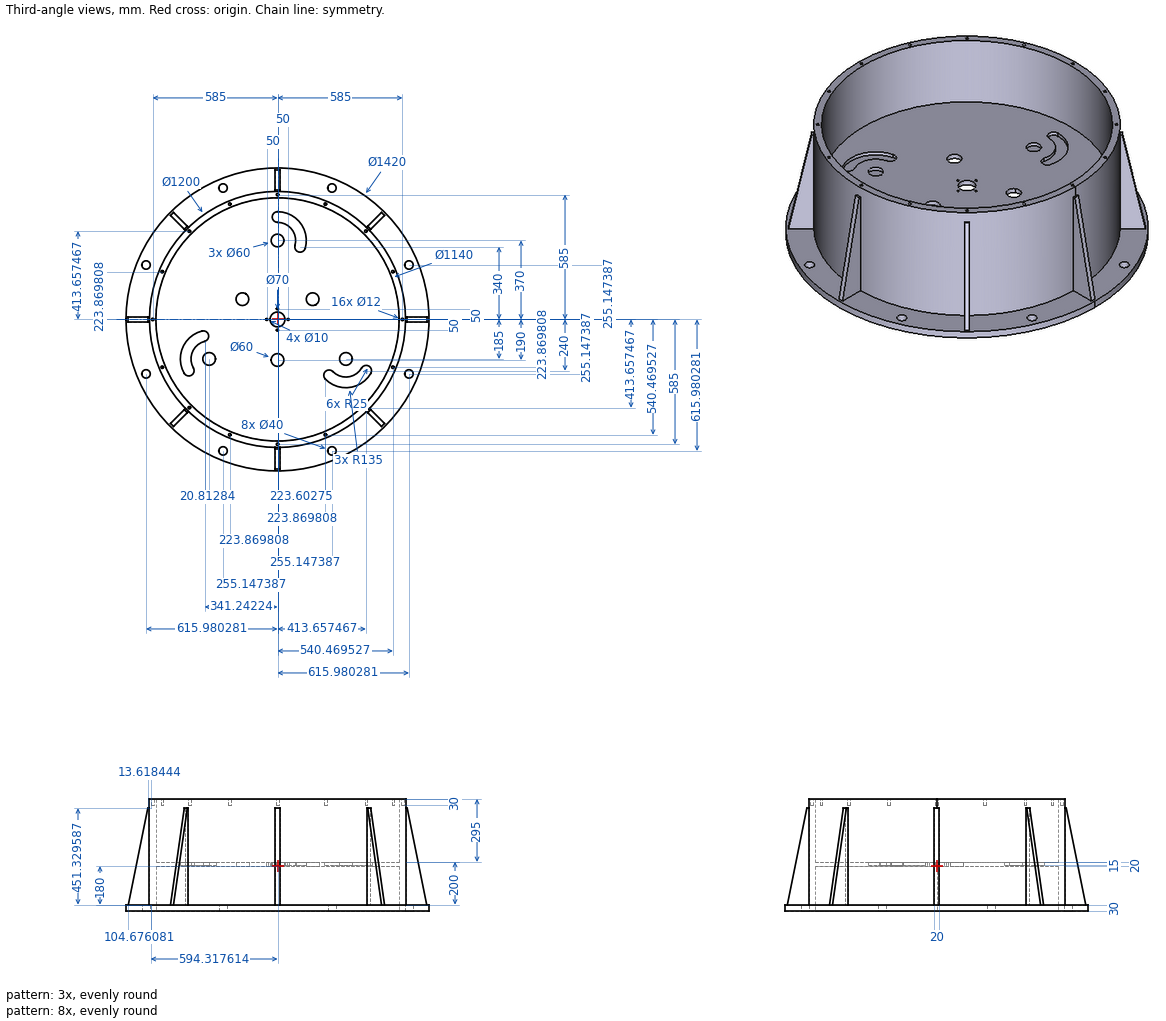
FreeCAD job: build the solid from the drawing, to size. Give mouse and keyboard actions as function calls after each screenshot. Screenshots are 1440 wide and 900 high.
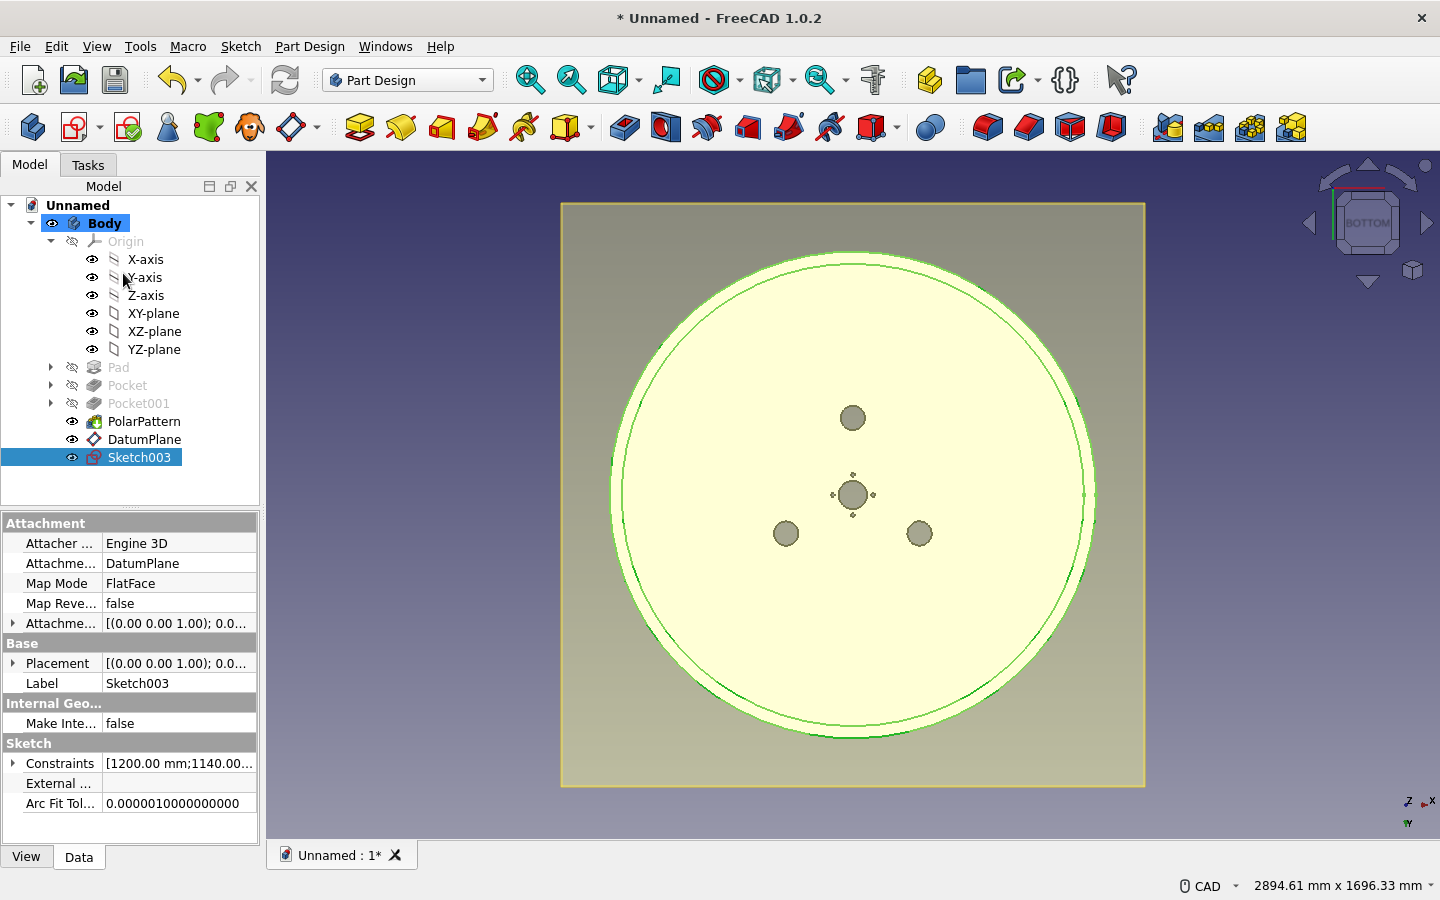
click(360, 128)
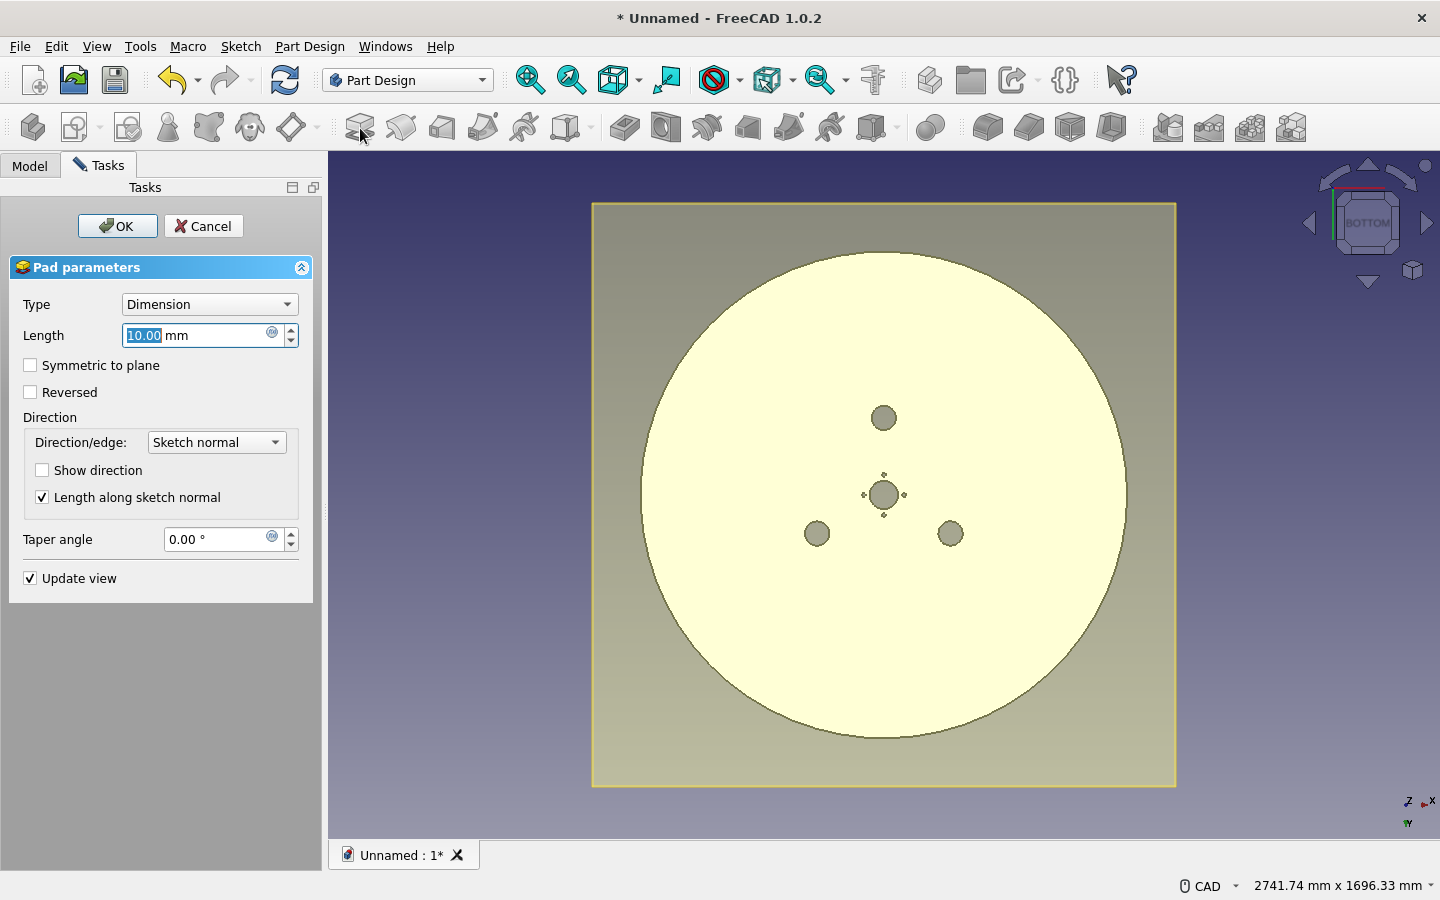
text(200)
key(Tab)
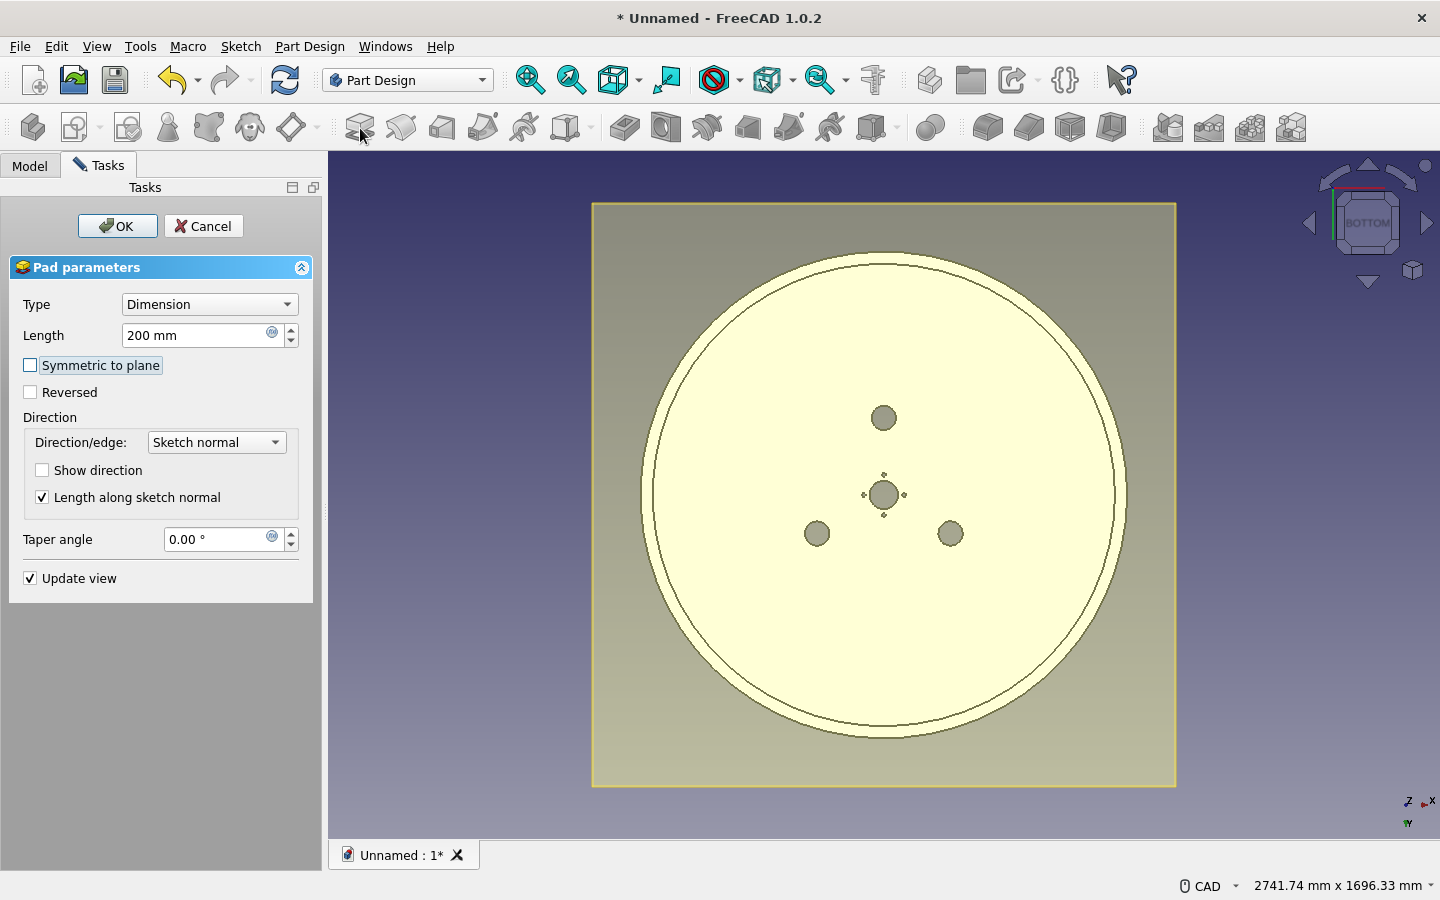
click(118, 226)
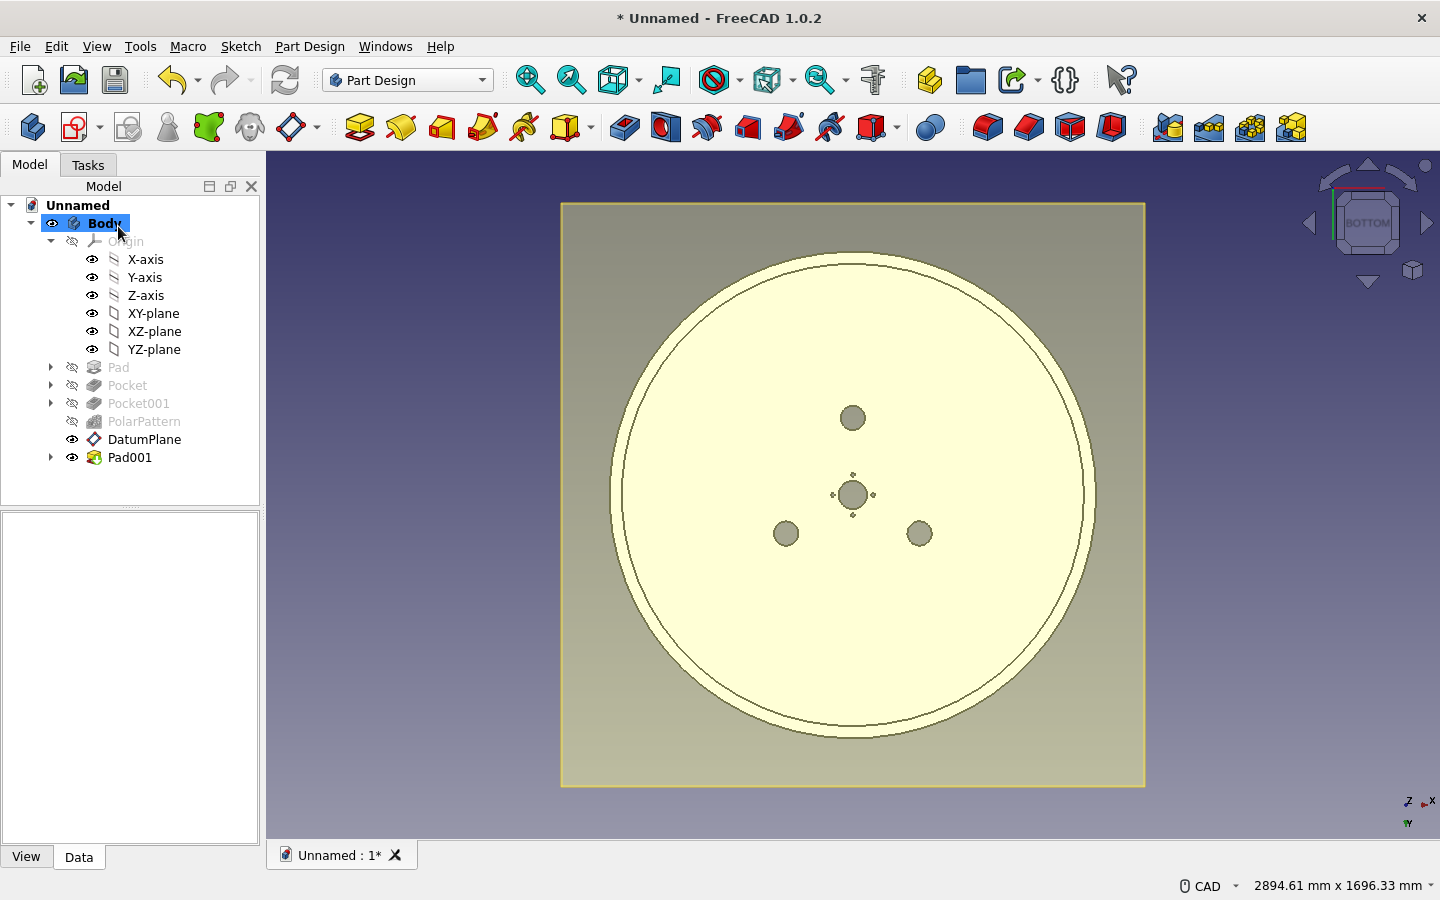
click(117, 439)
key(space)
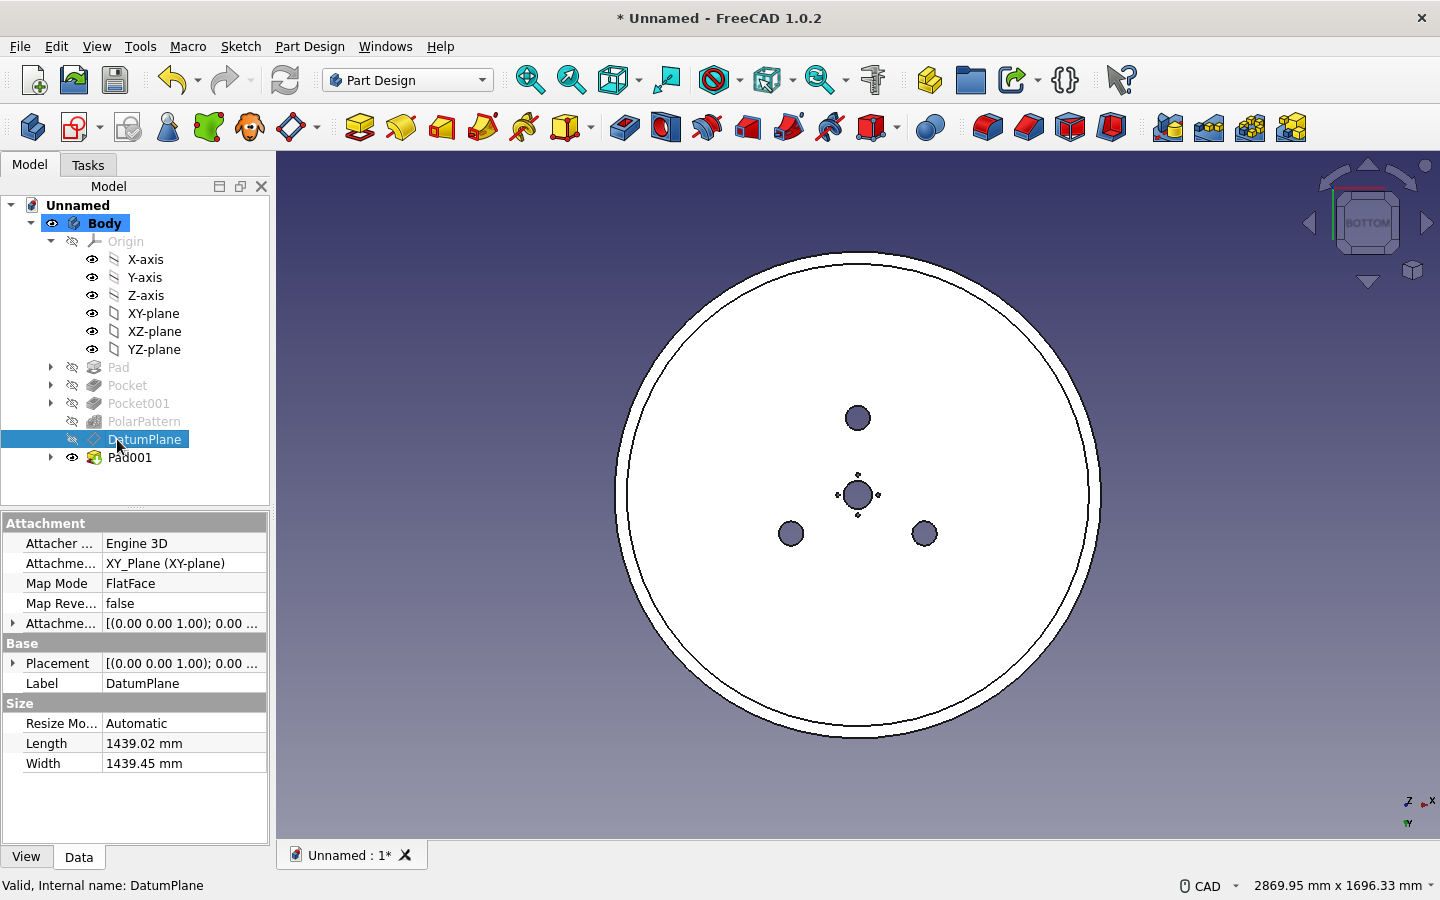
key(0)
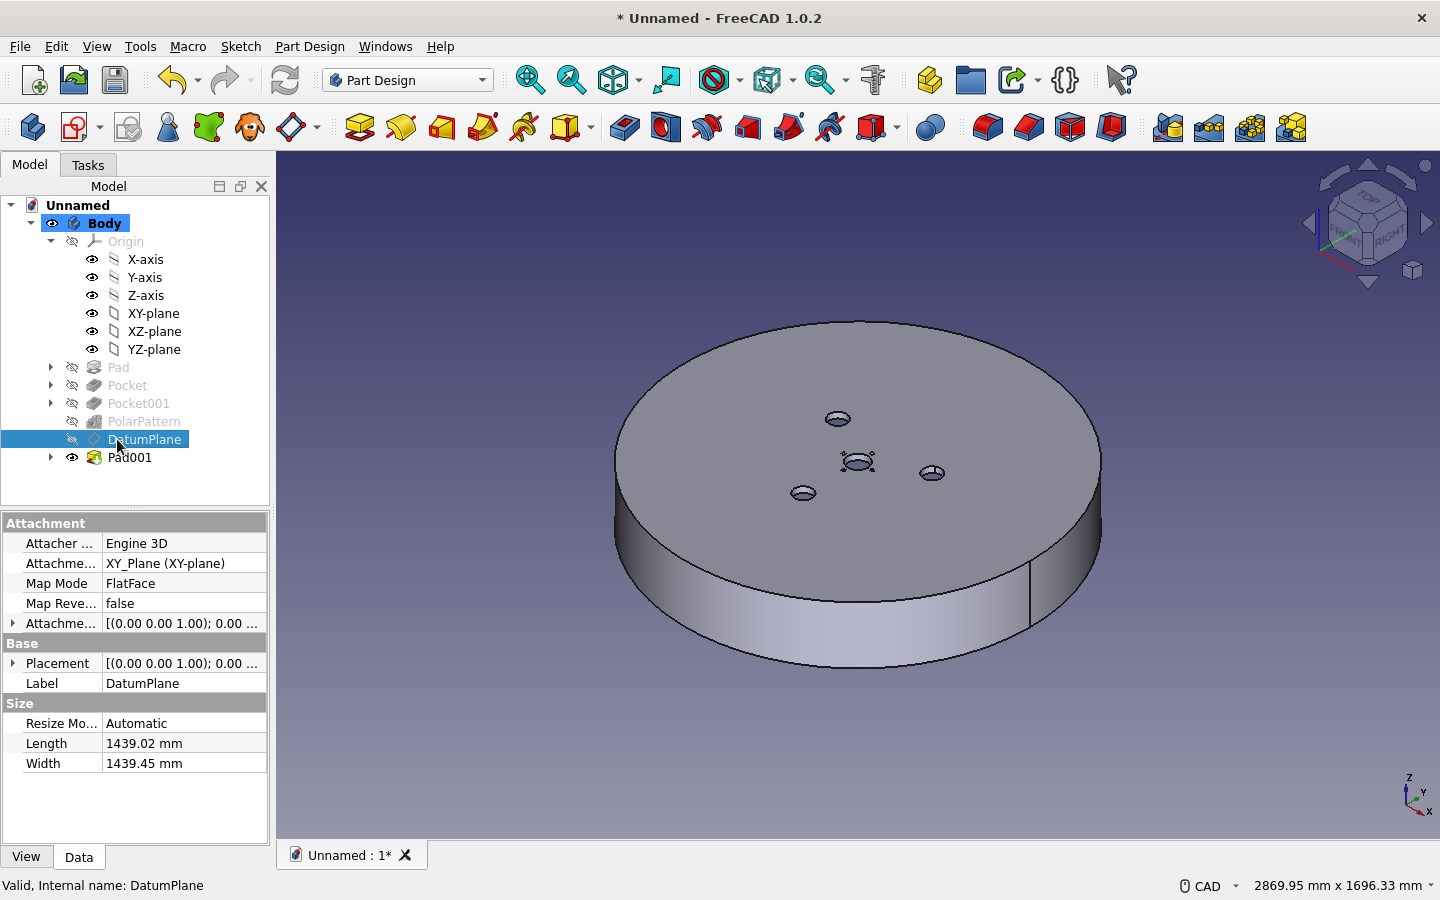
click(956, 404)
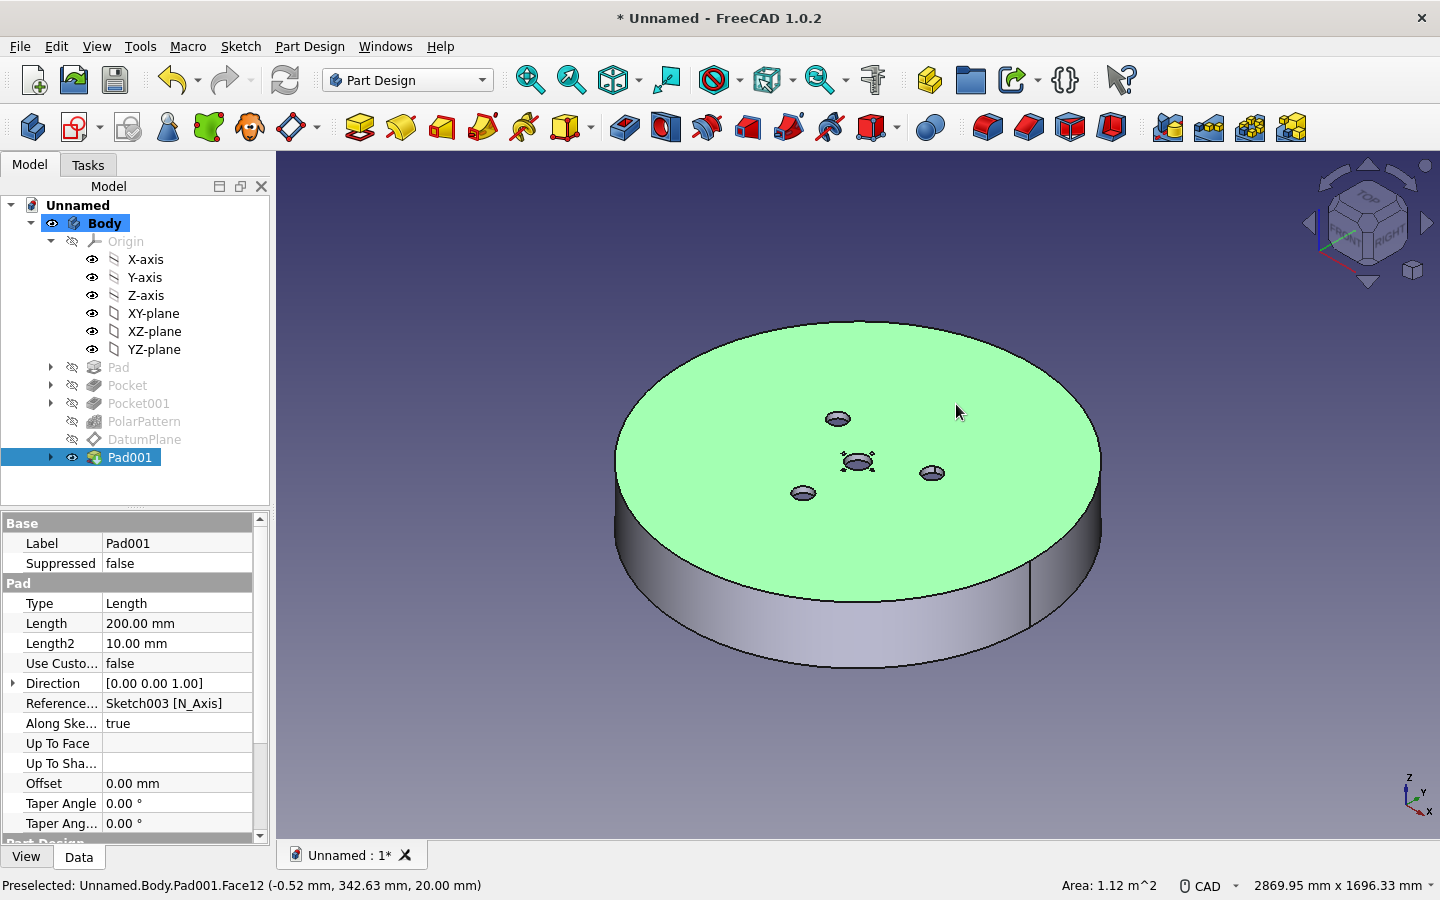
click(74, 128)